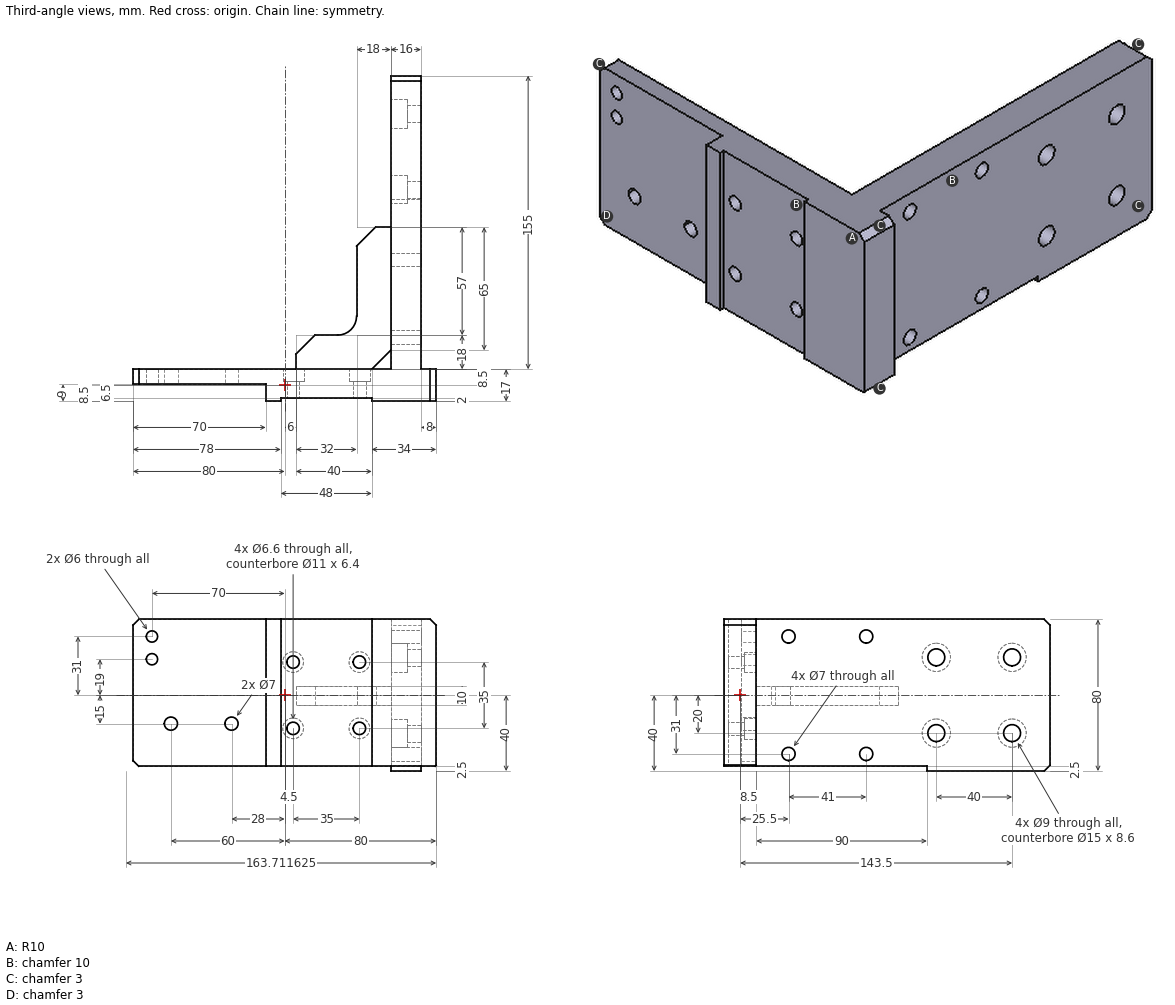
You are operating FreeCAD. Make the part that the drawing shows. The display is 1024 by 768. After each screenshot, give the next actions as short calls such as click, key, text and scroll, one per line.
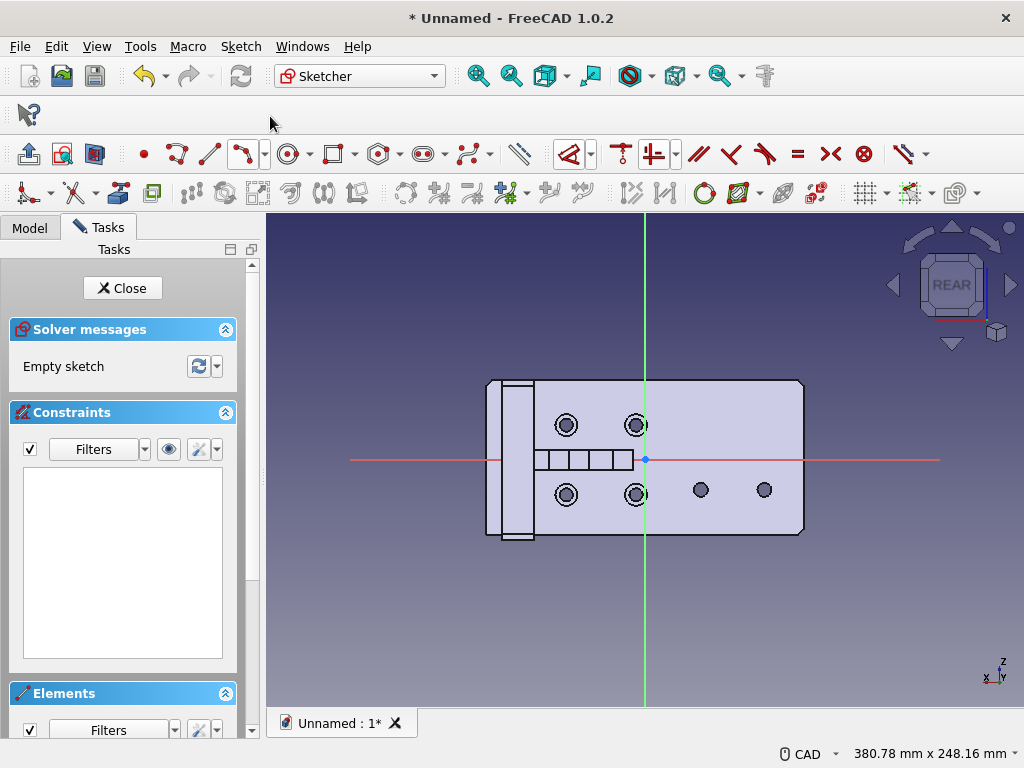
scroll(810, 404, up, 11)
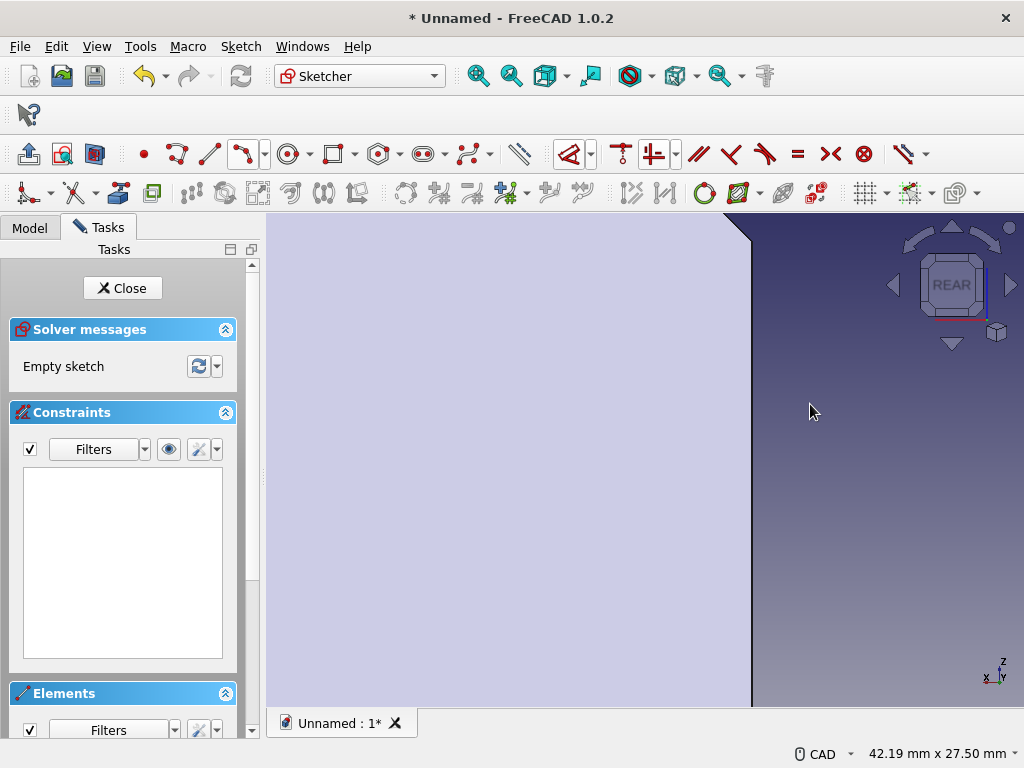
click(288, 154)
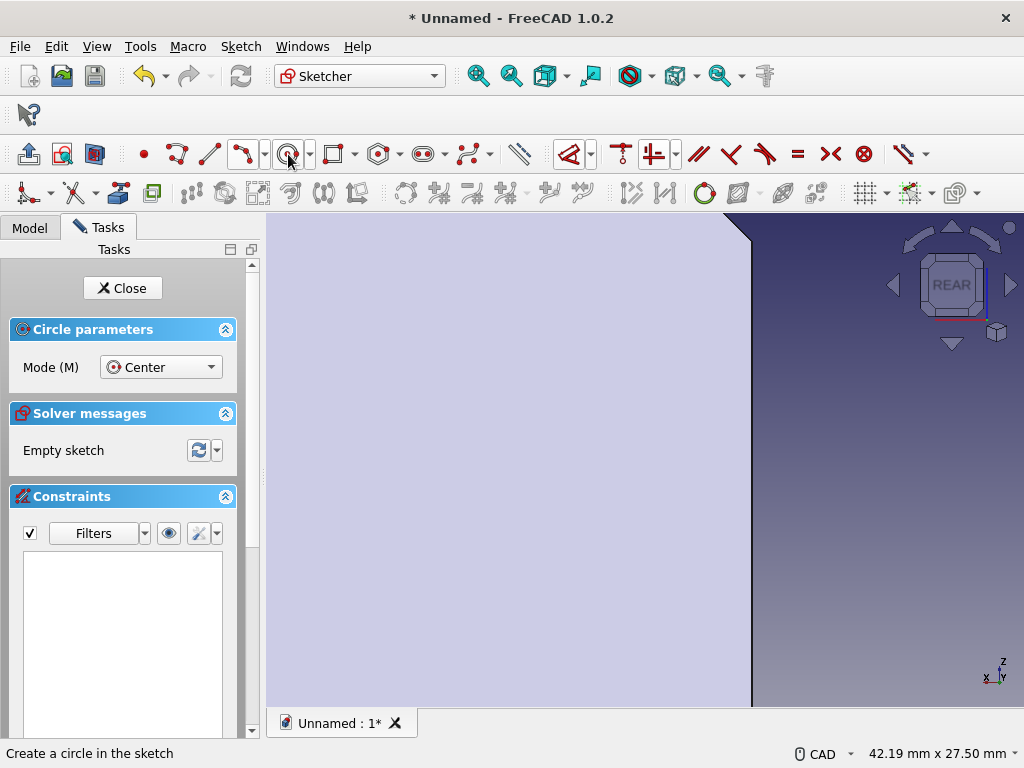
click(573, 349)
click(611, 311)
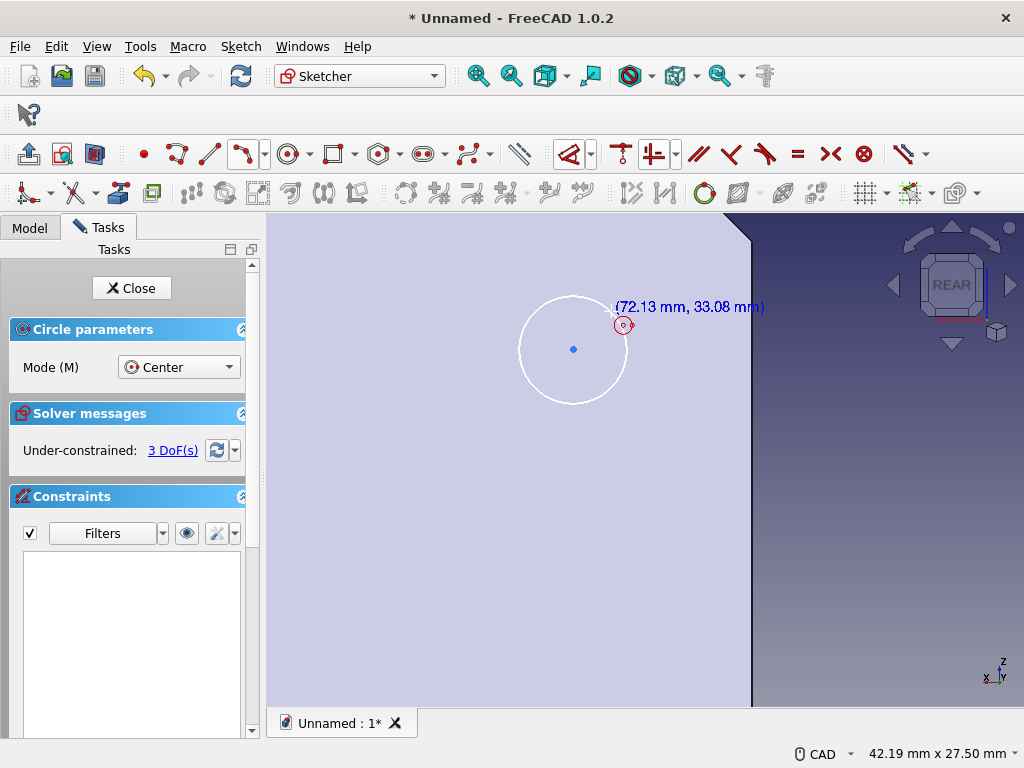
click(573, 565)
click(611, 527)
key(Escape)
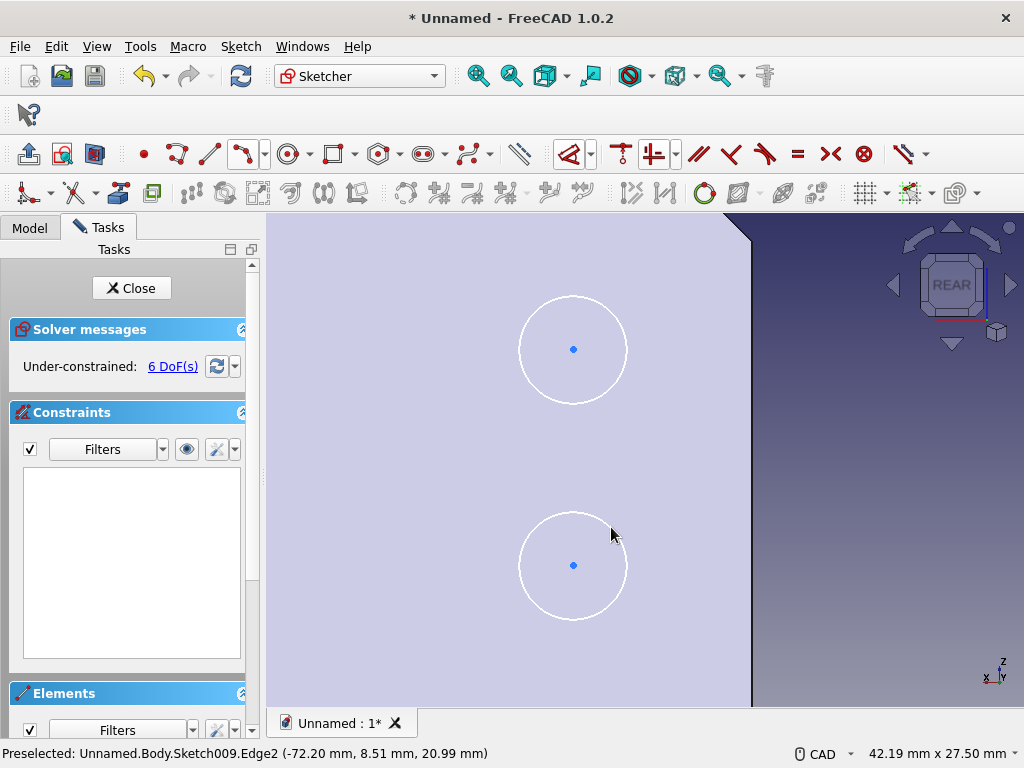
click(611, 312)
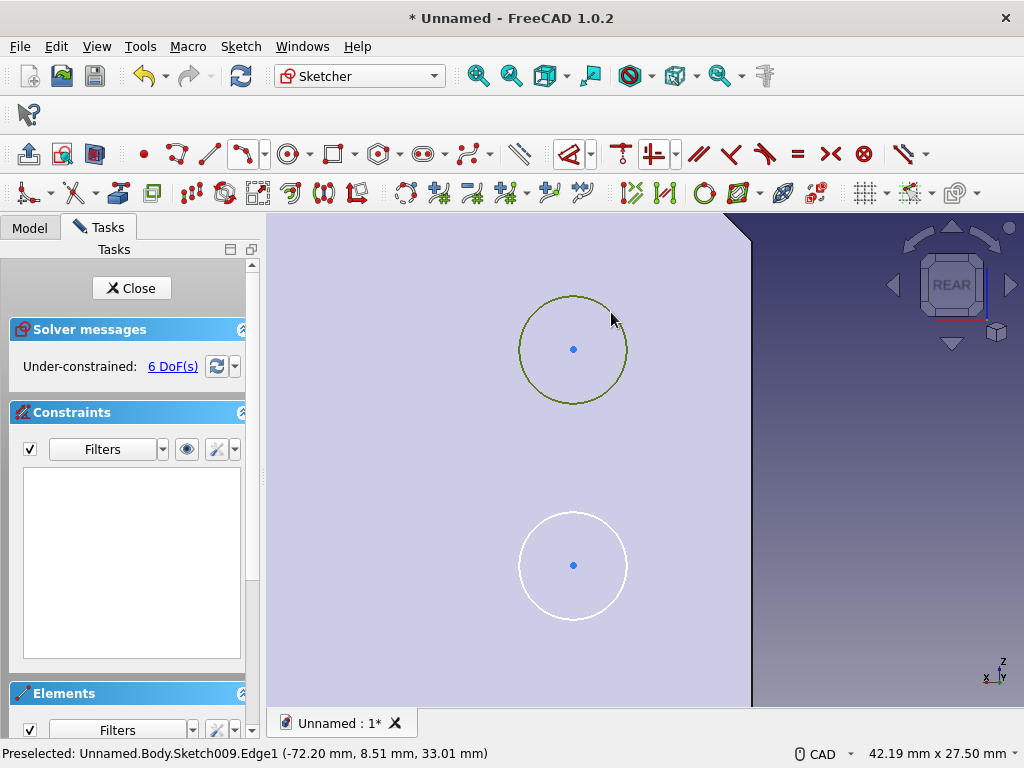
click(611, 528)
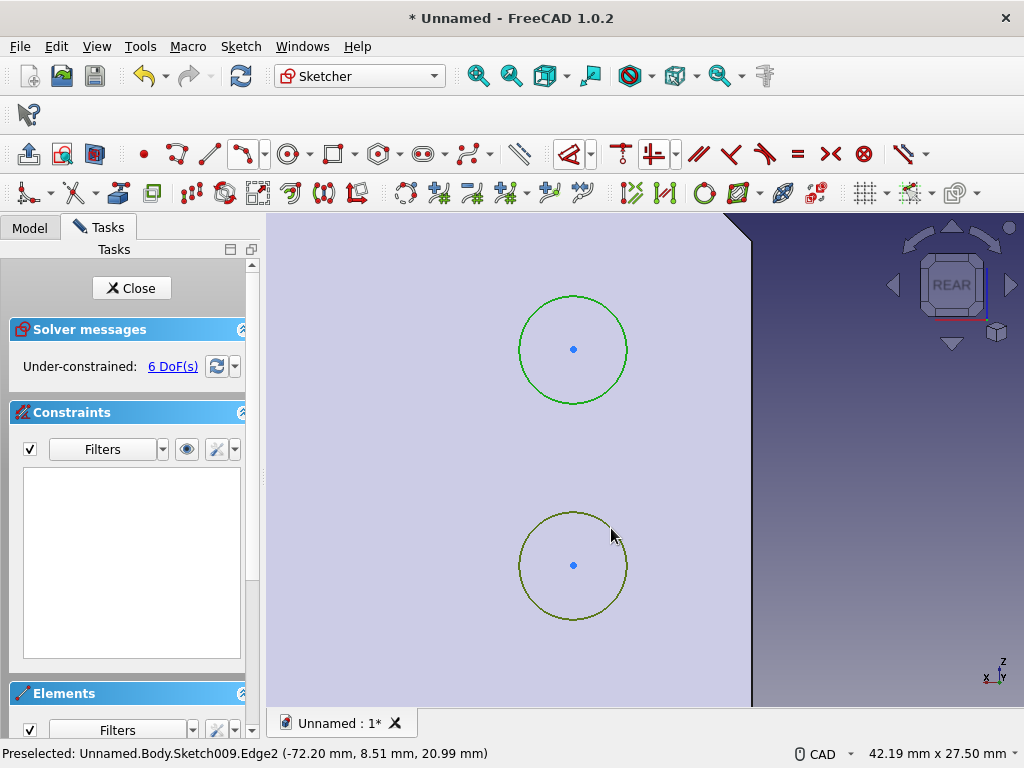
click(798, 154)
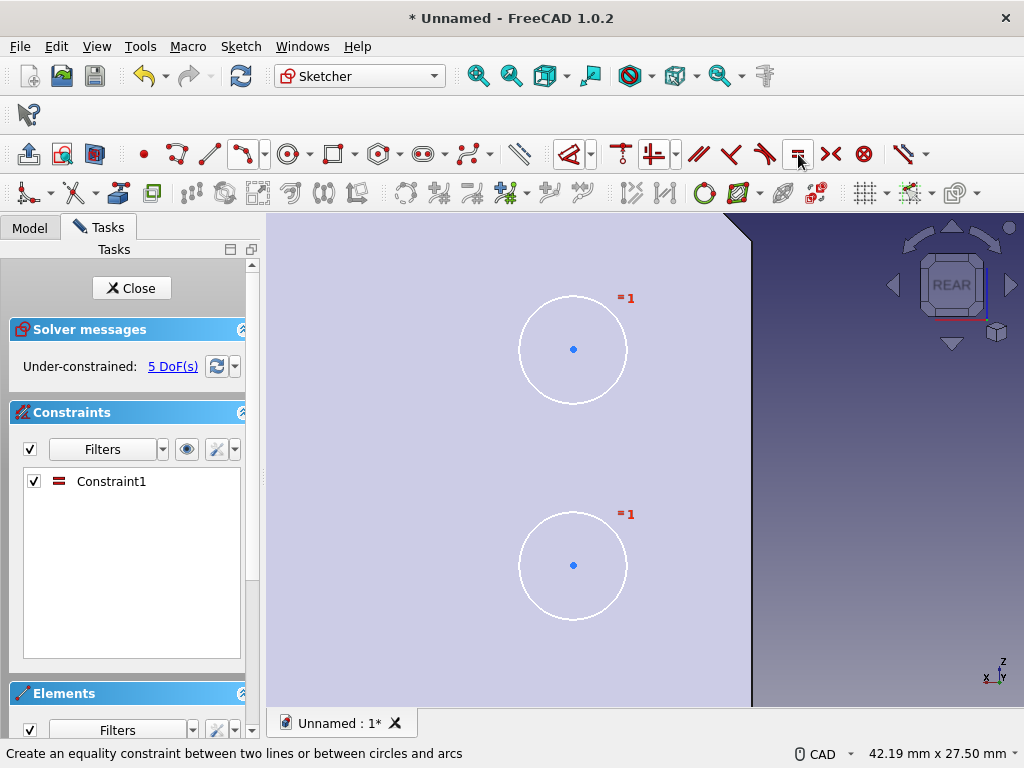
click(611, 312)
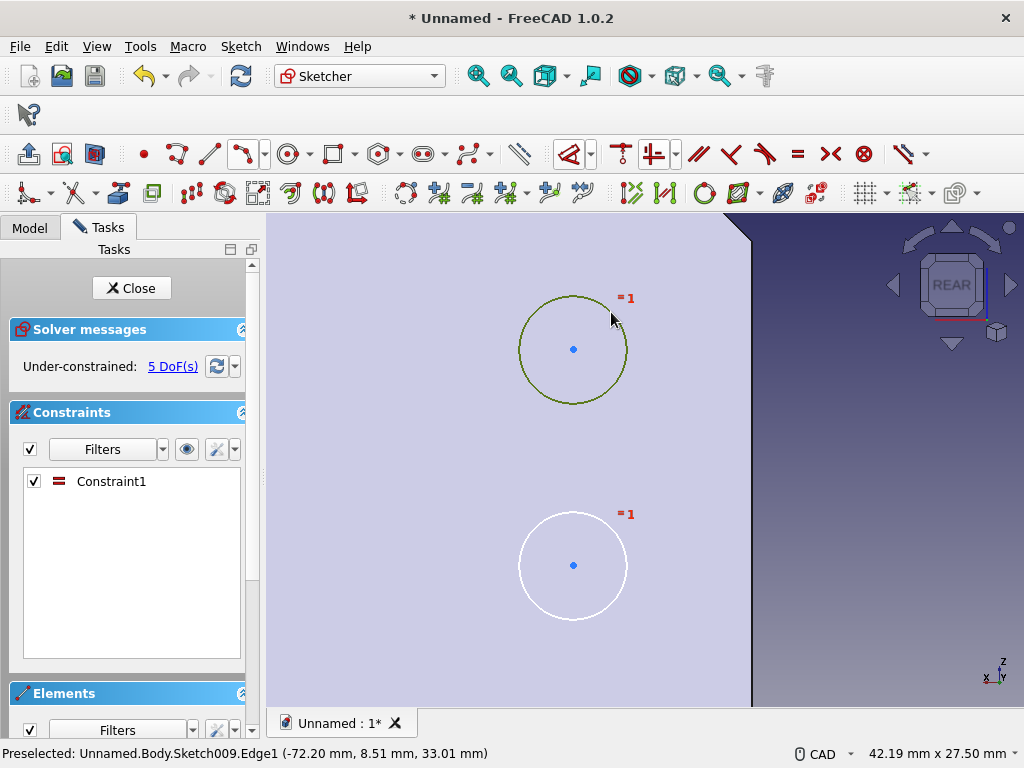
click(590, 154)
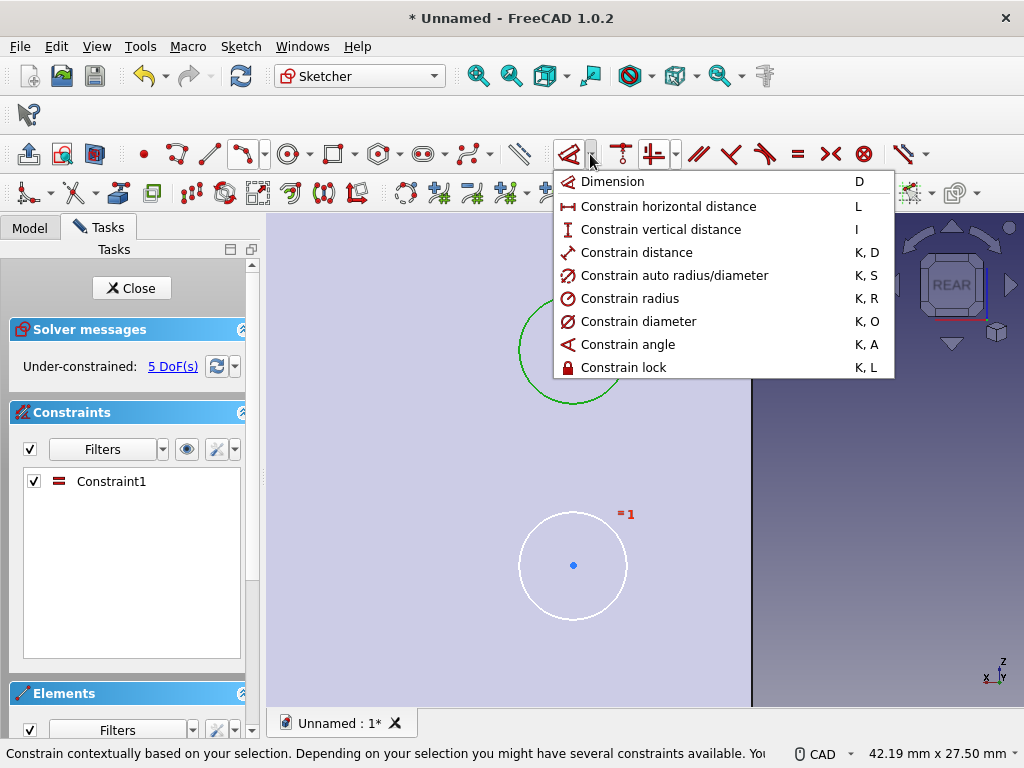
click(724, 322)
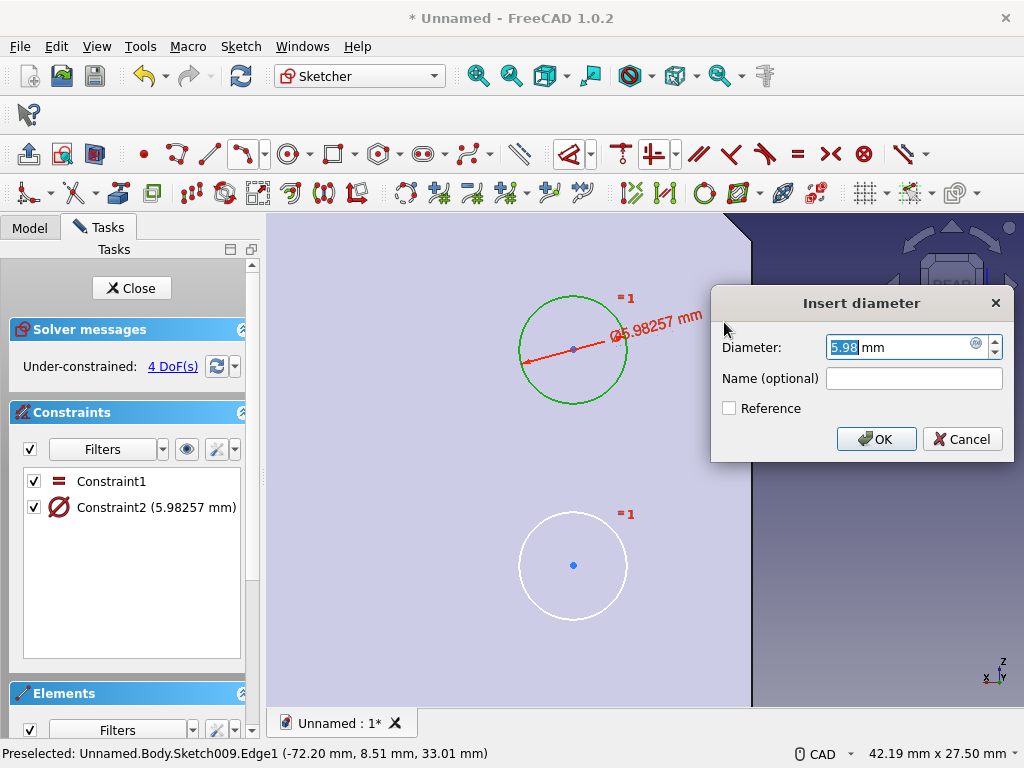
text(6)
key(Return)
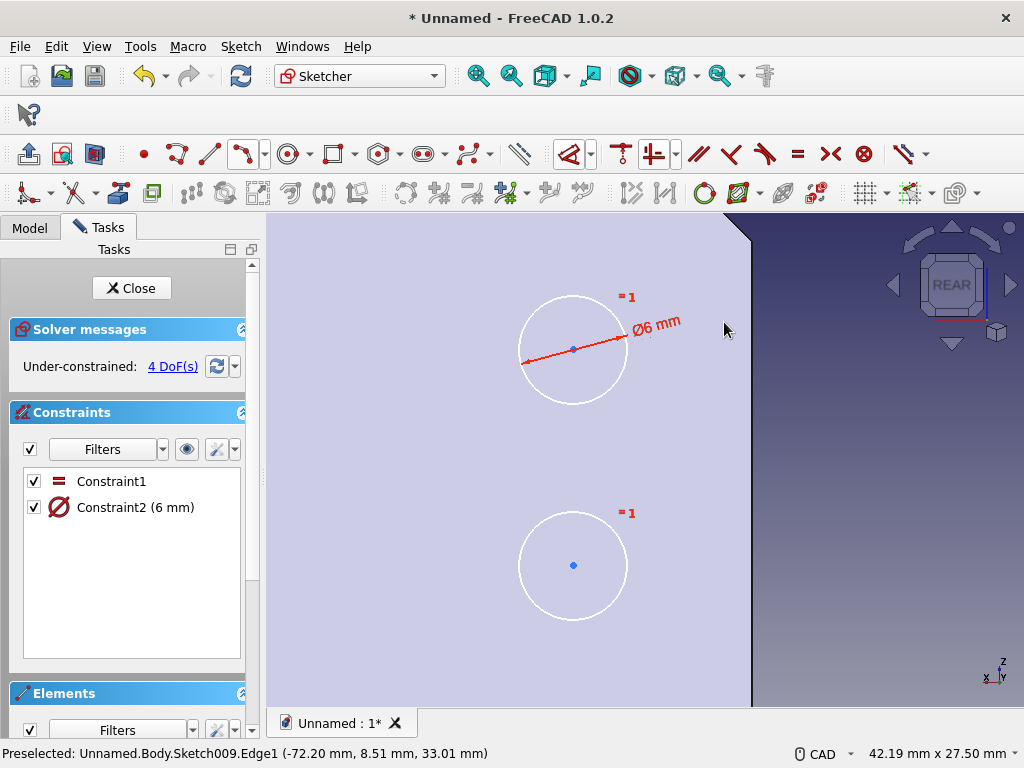
click(573, 350)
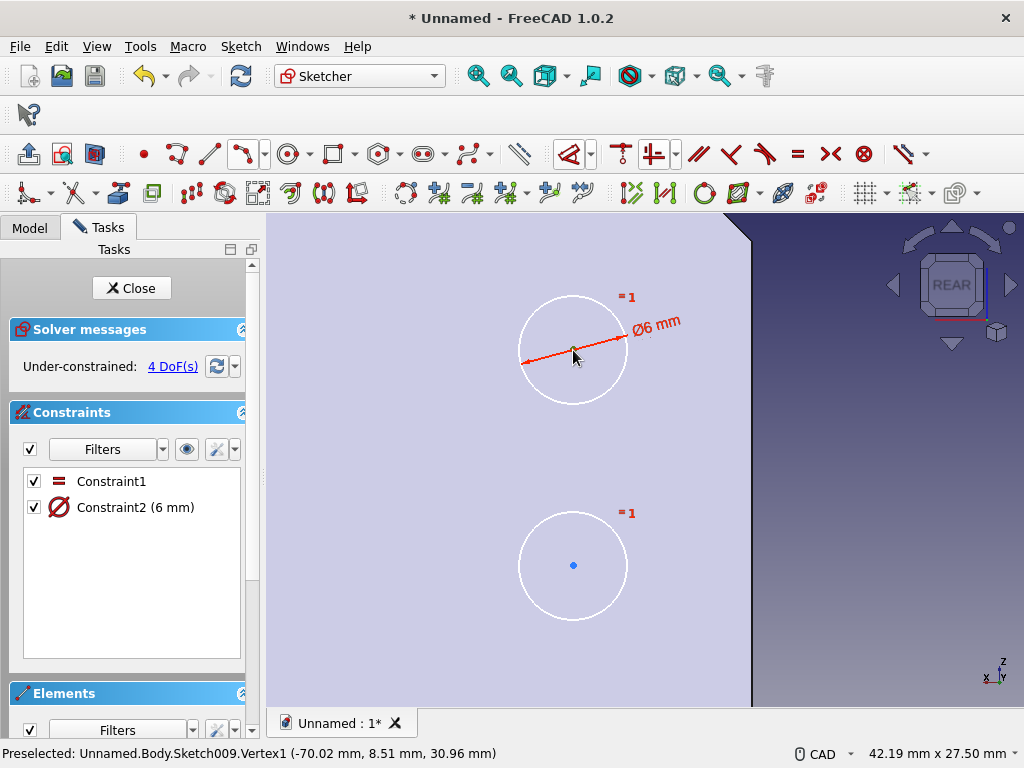
key(l)